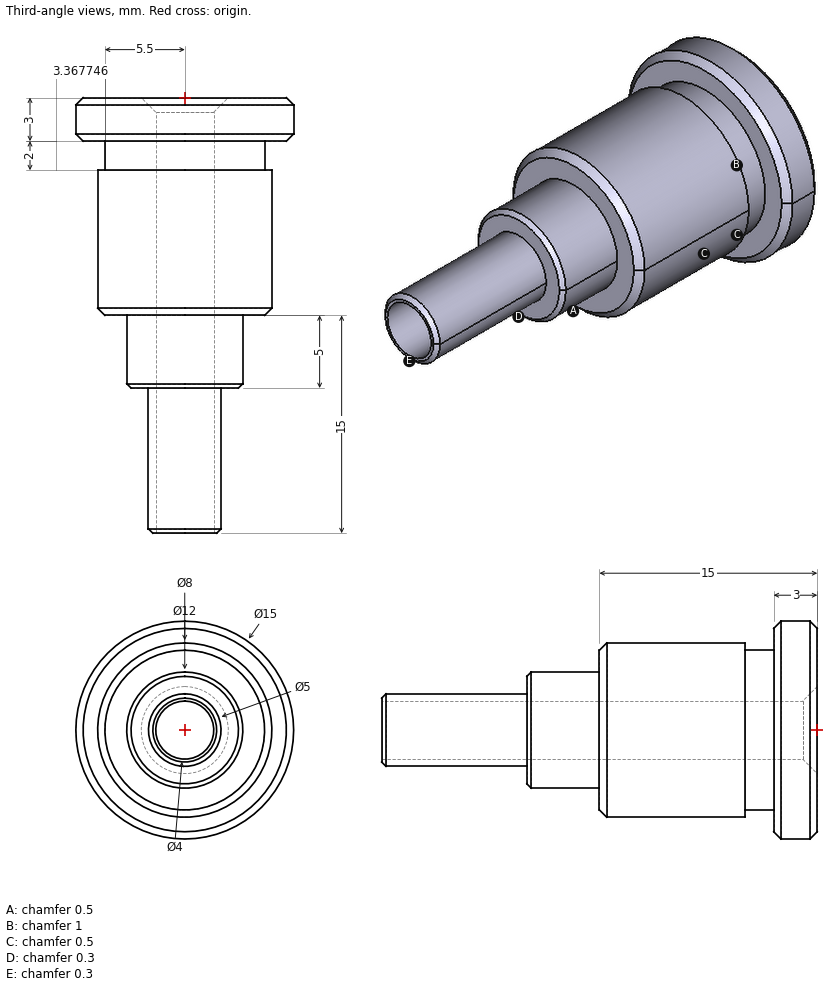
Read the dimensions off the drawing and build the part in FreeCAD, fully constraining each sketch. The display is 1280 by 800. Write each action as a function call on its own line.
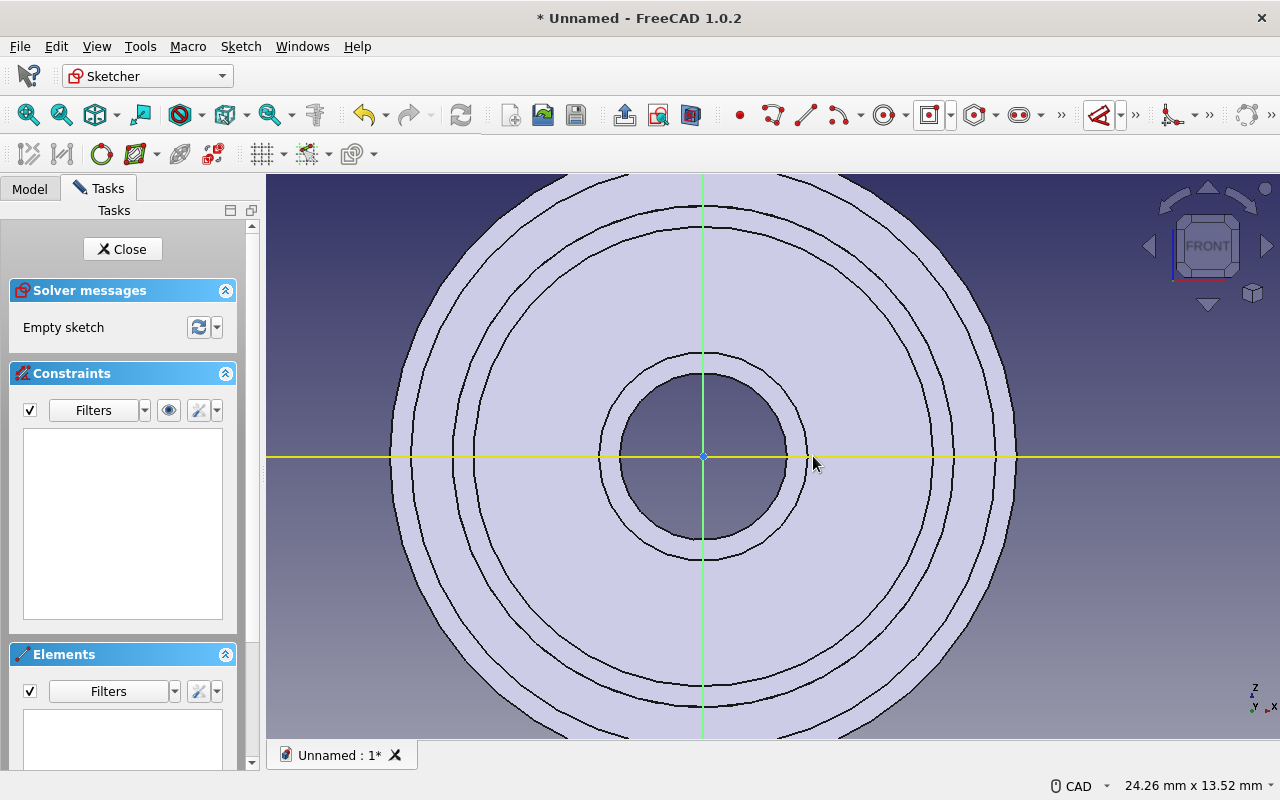
click(884, 116)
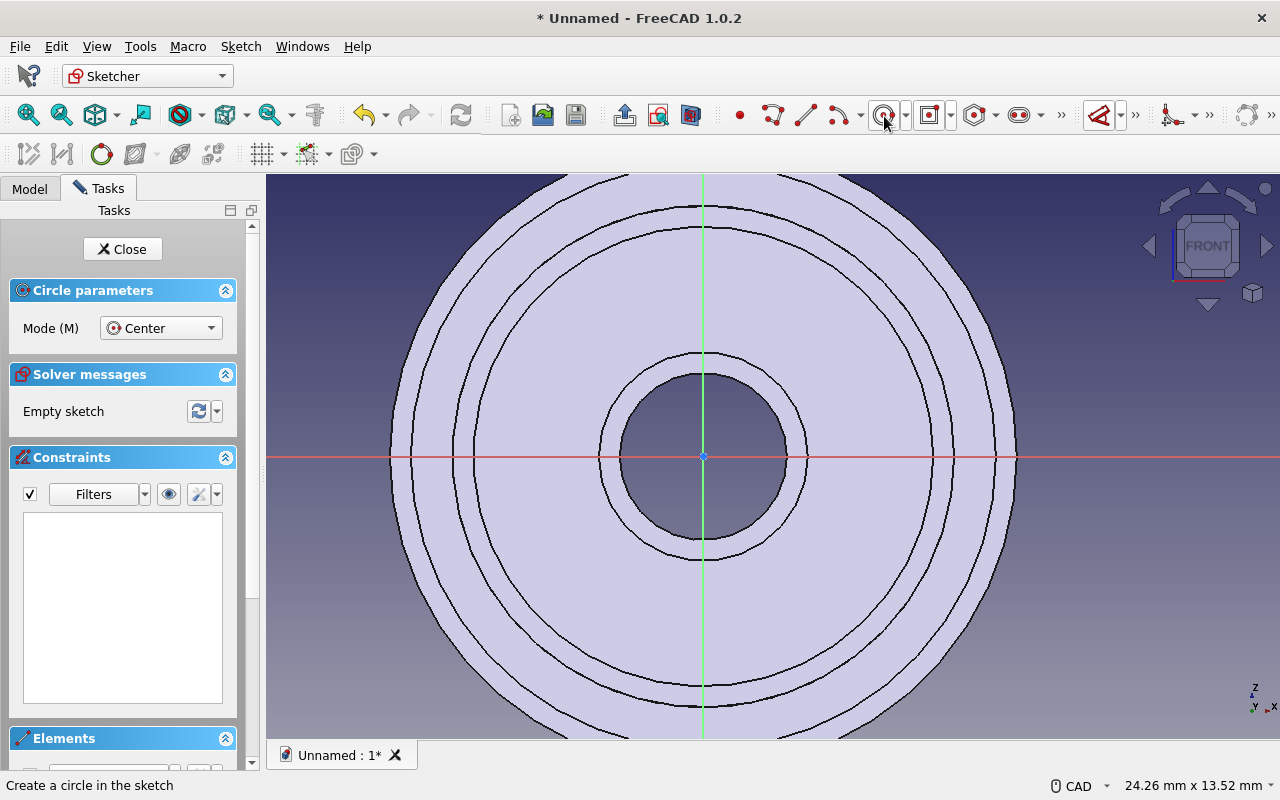
click(703, 456)
move(822, 338)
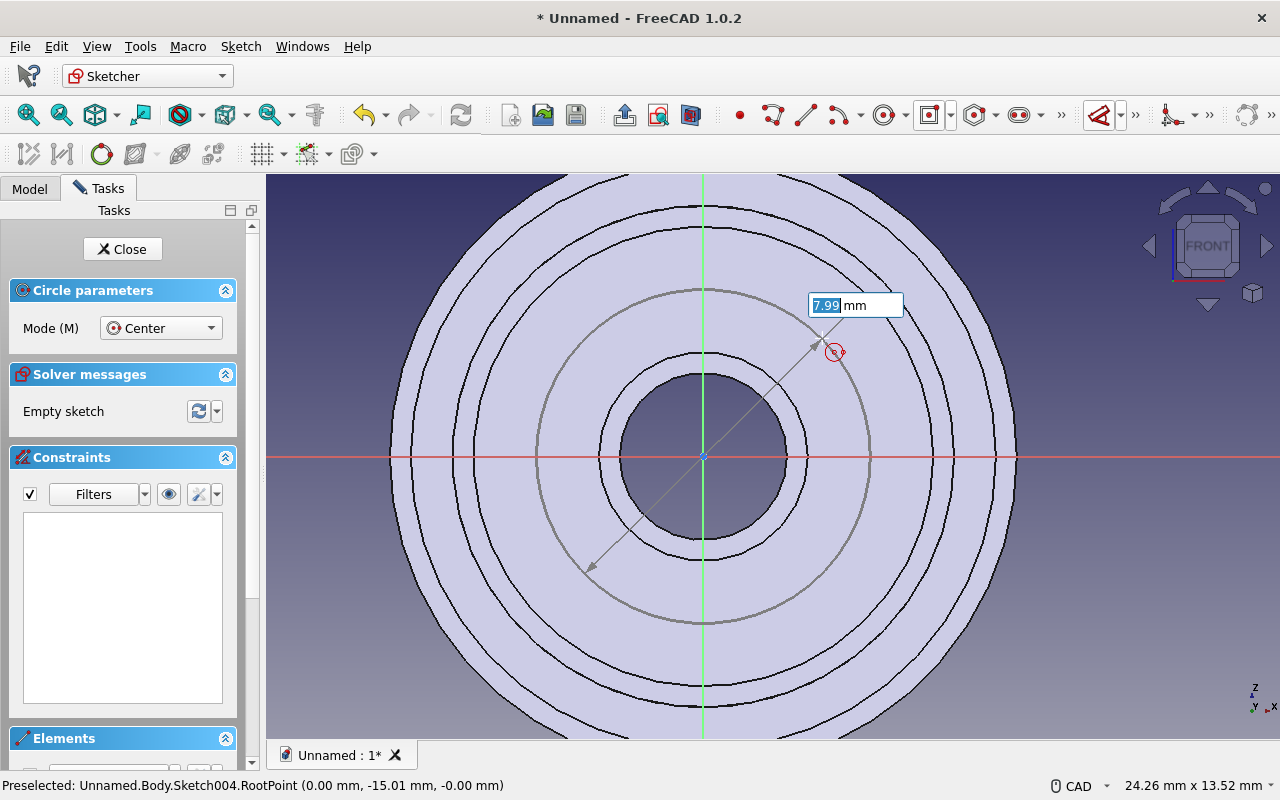
text(8)
key(Return)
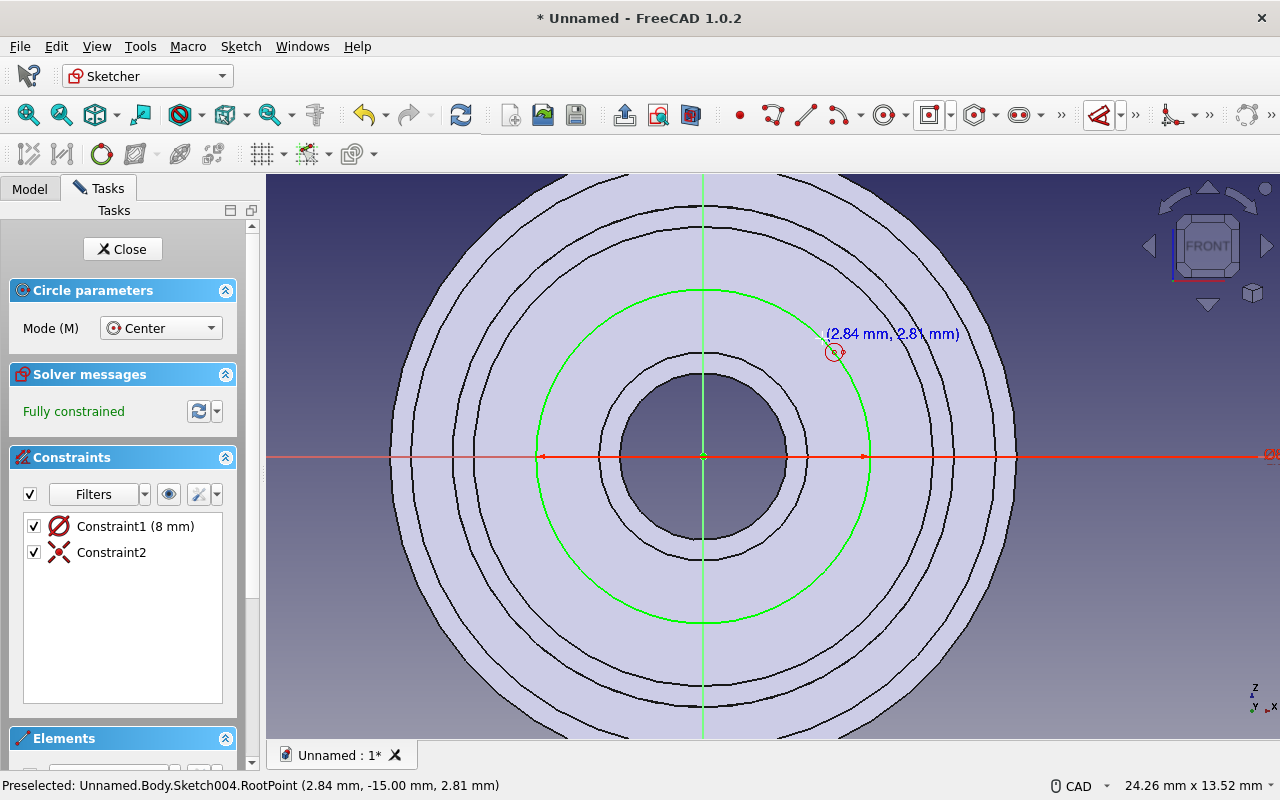
click(703, 456)
move(777, 383)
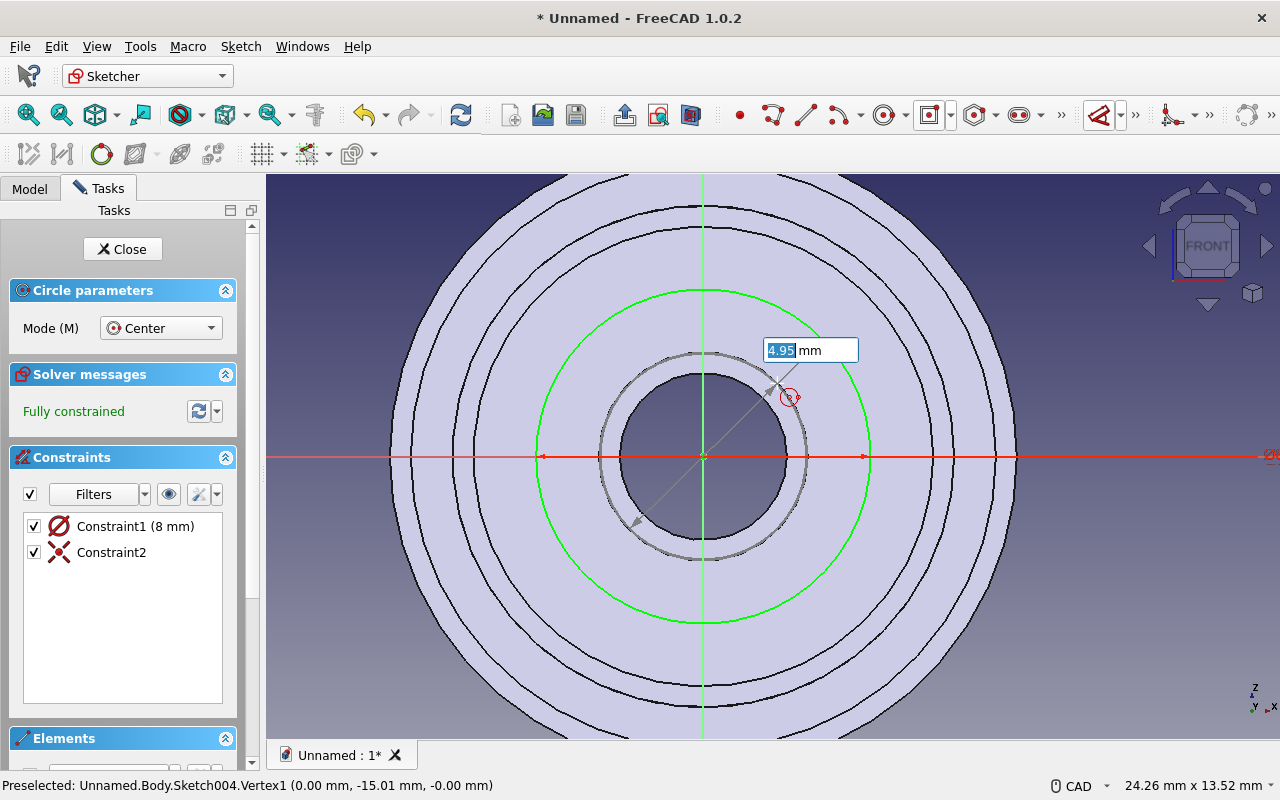
text(5)
key(Return)
key(Escape)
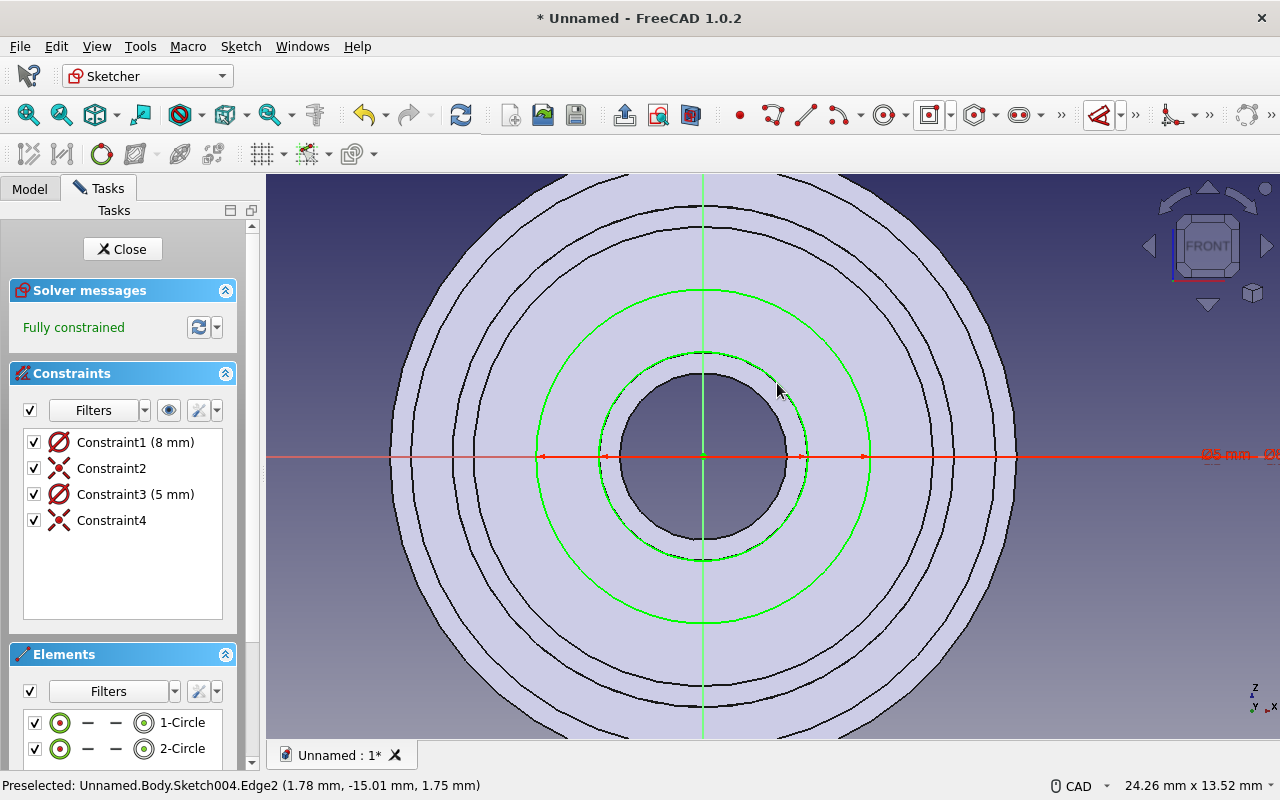
click(123, 249)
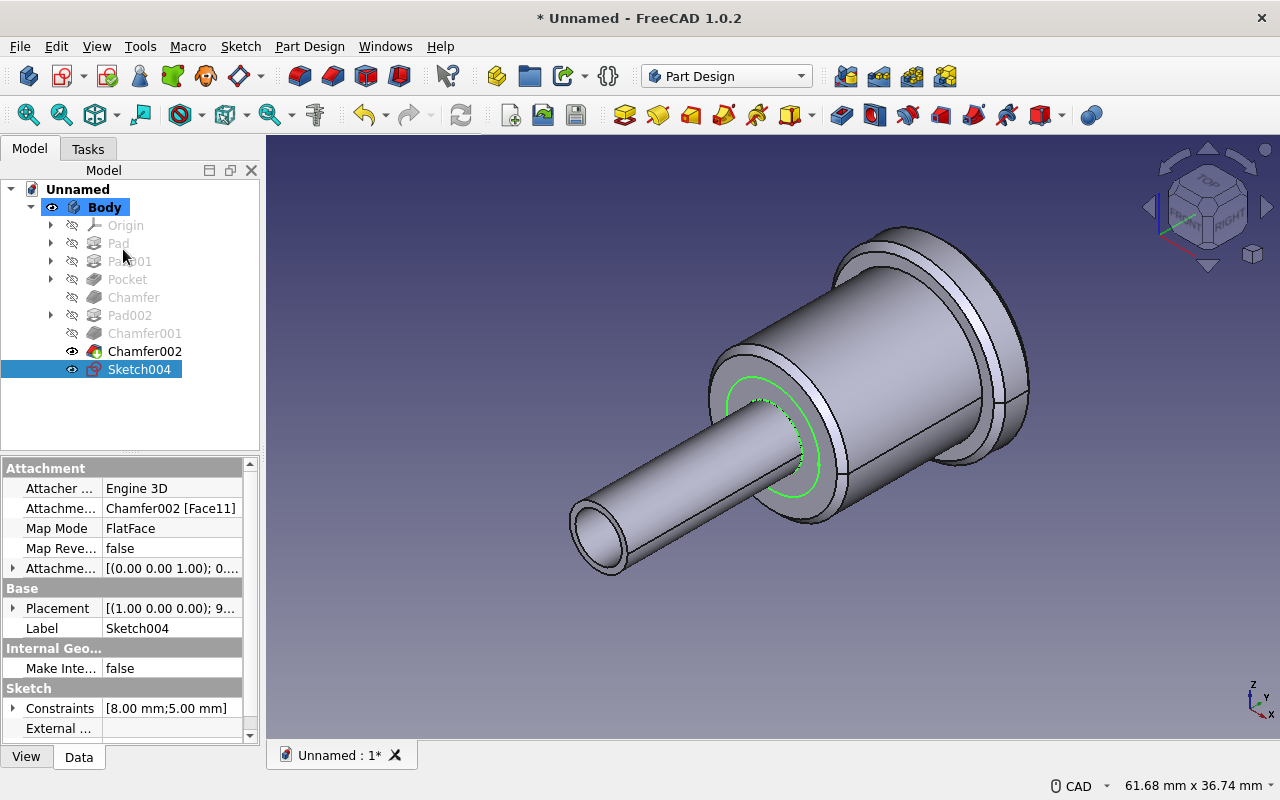
click(625, 116)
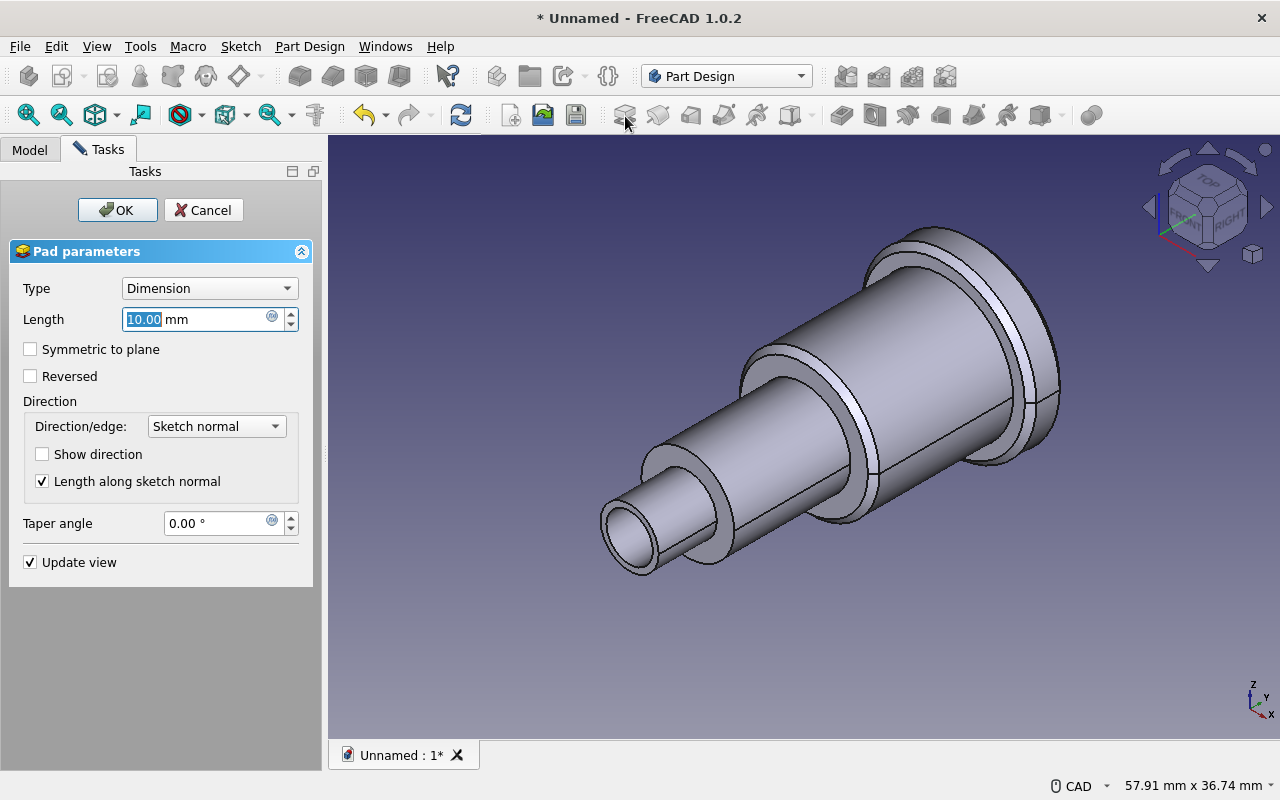
text(5)
key(Tab)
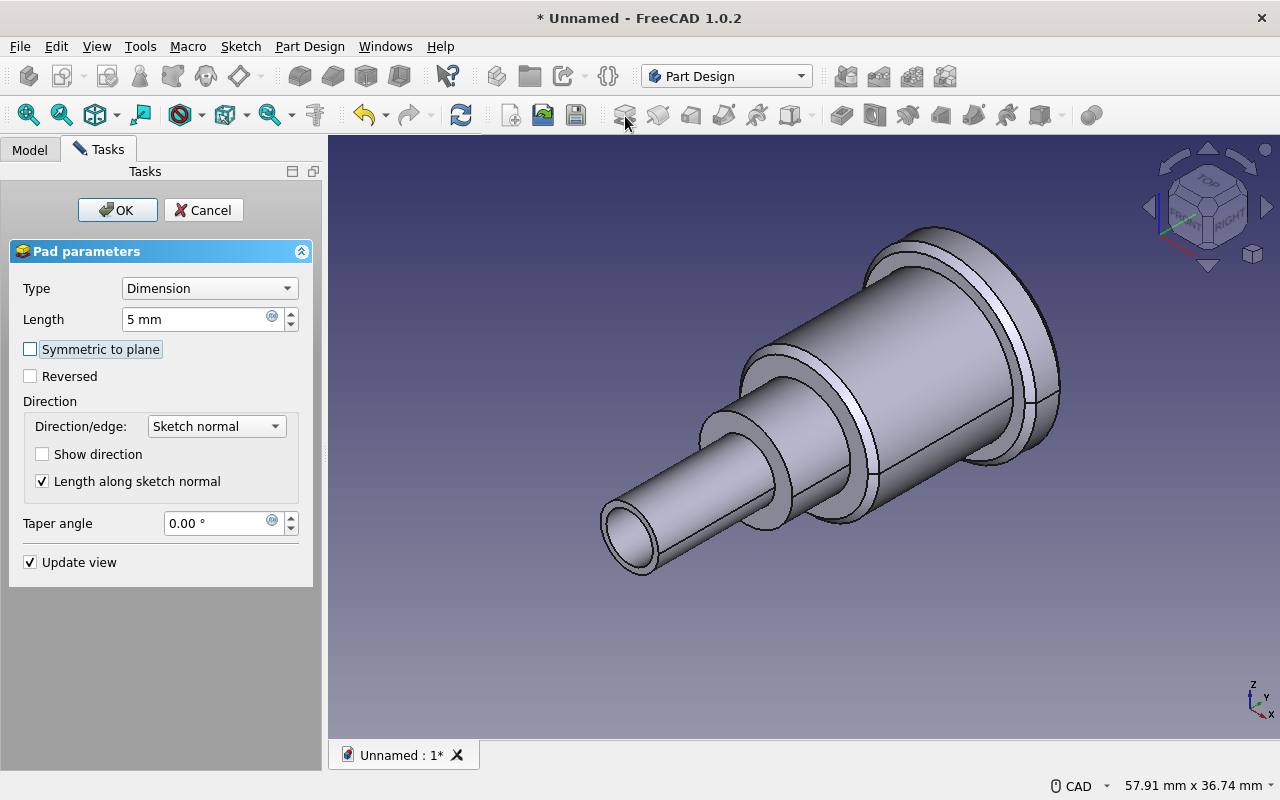
click(118, 210)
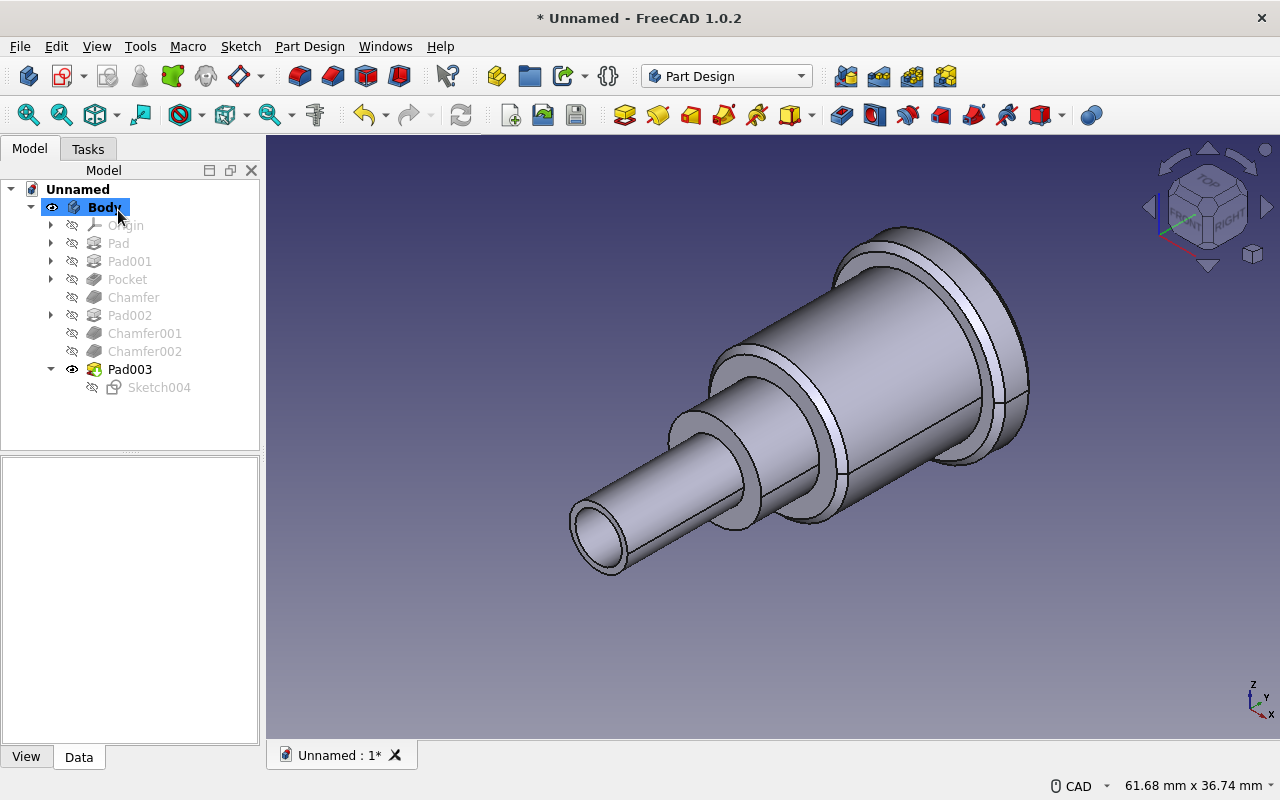
click(701, 410)